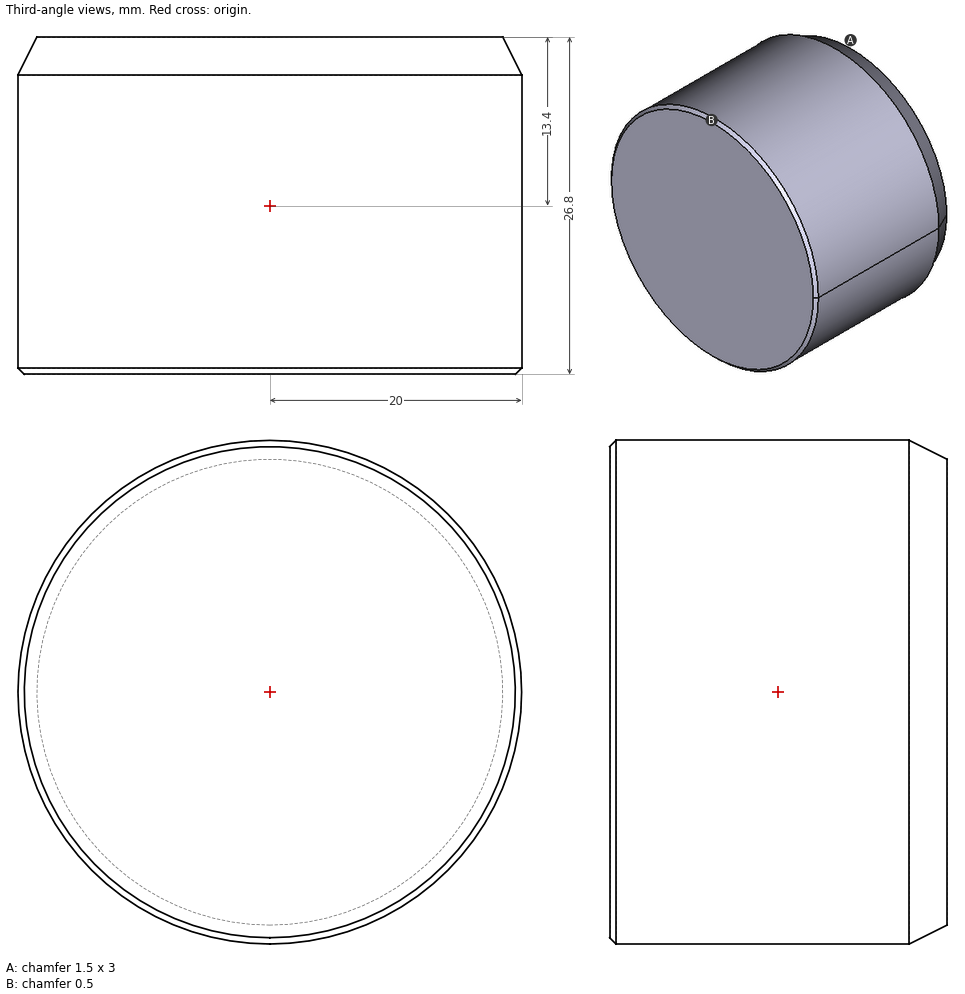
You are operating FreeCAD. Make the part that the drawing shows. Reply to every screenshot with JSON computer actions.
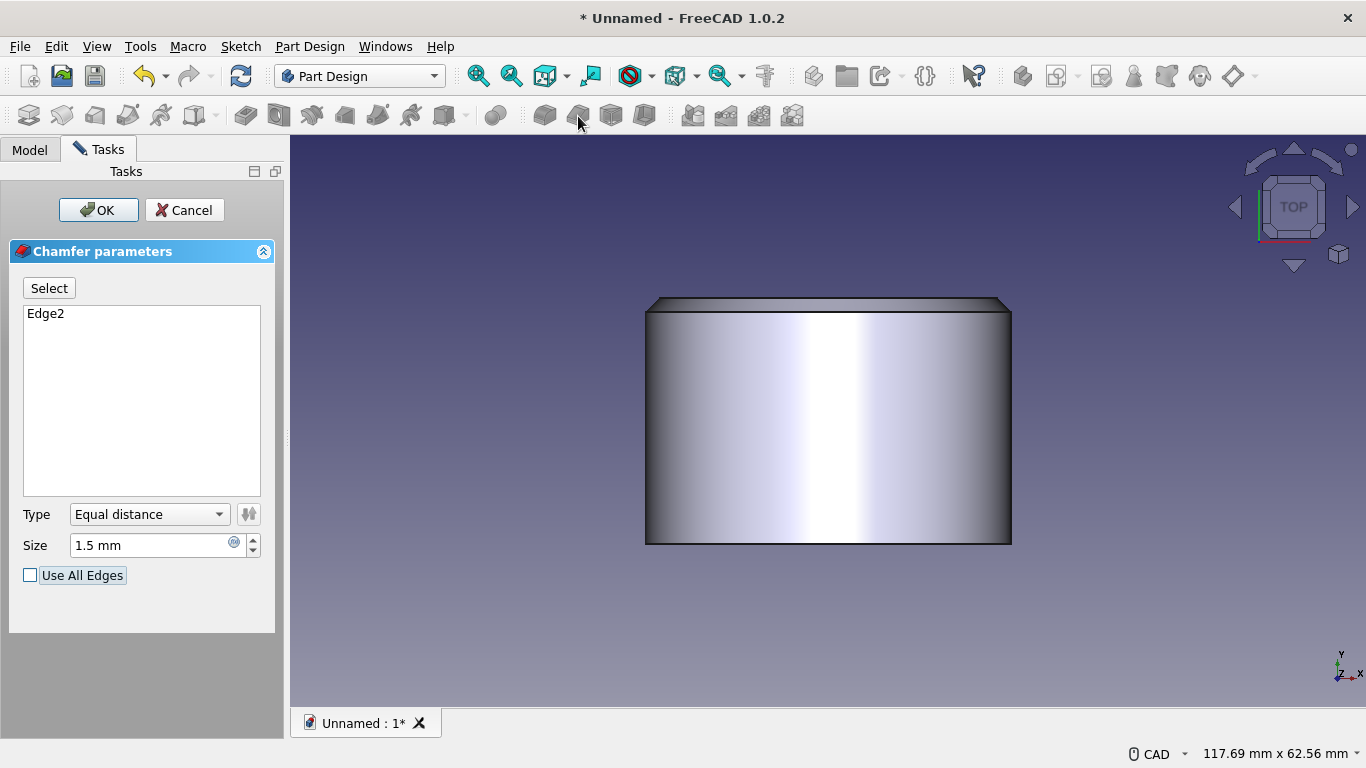
{"action": "left_click", "coordinate": [150, 514]}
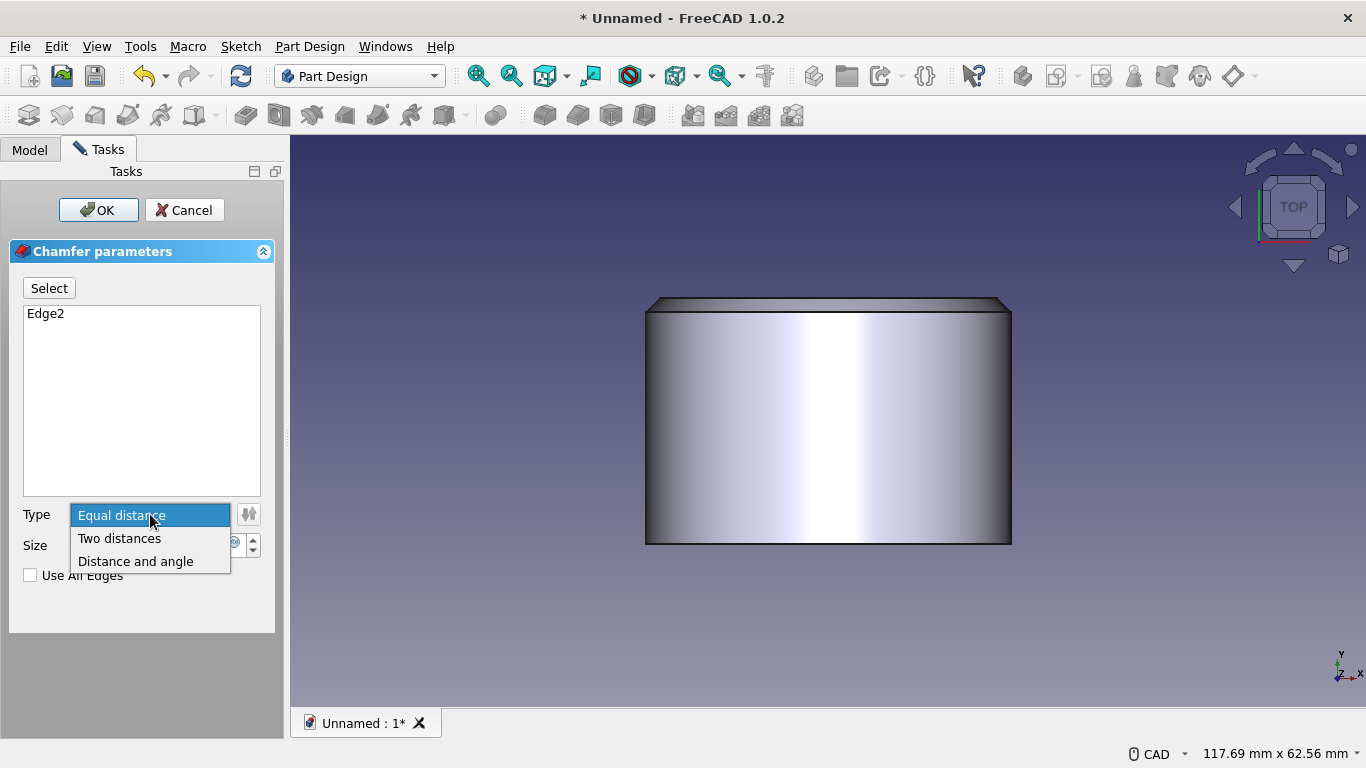
{"action": "left_click", "coordinate": [148, 538]}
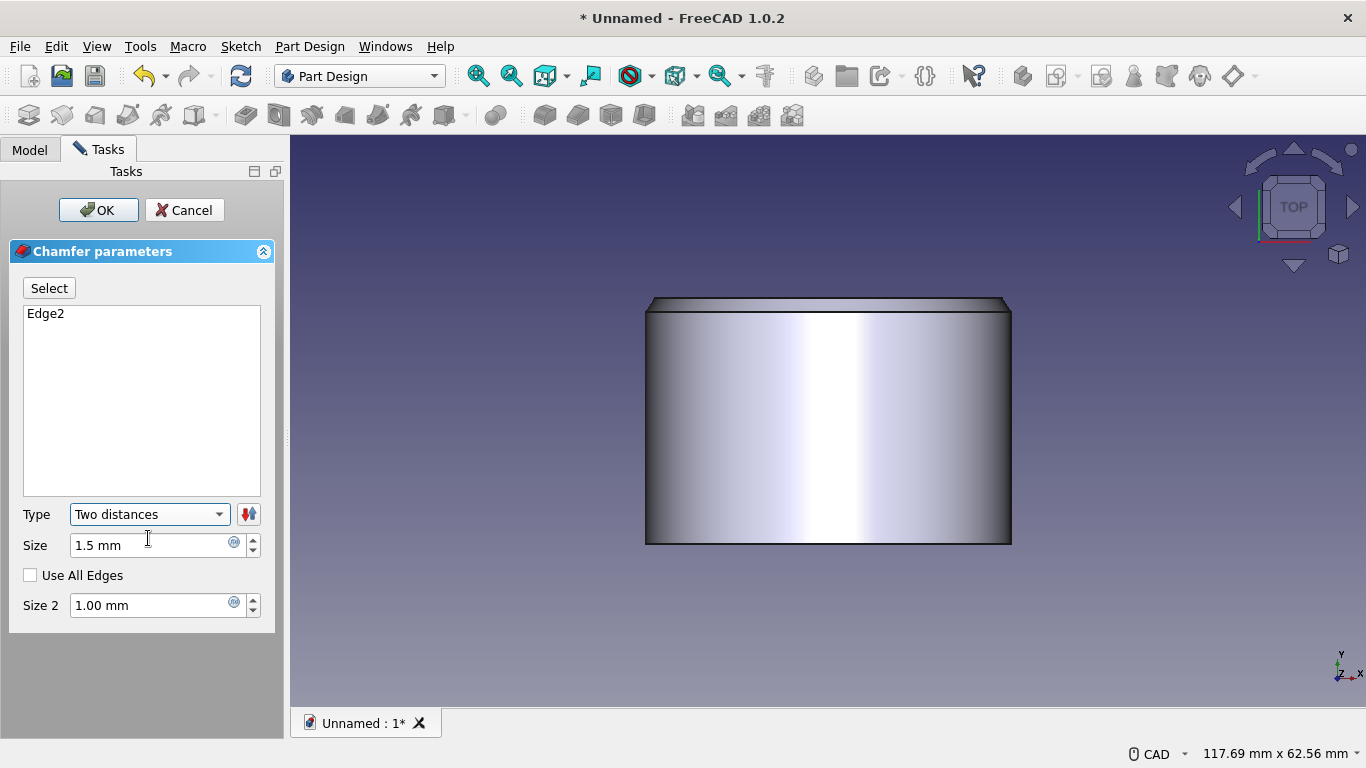
{"action": "triple_click", "coordinate": [158, 606]}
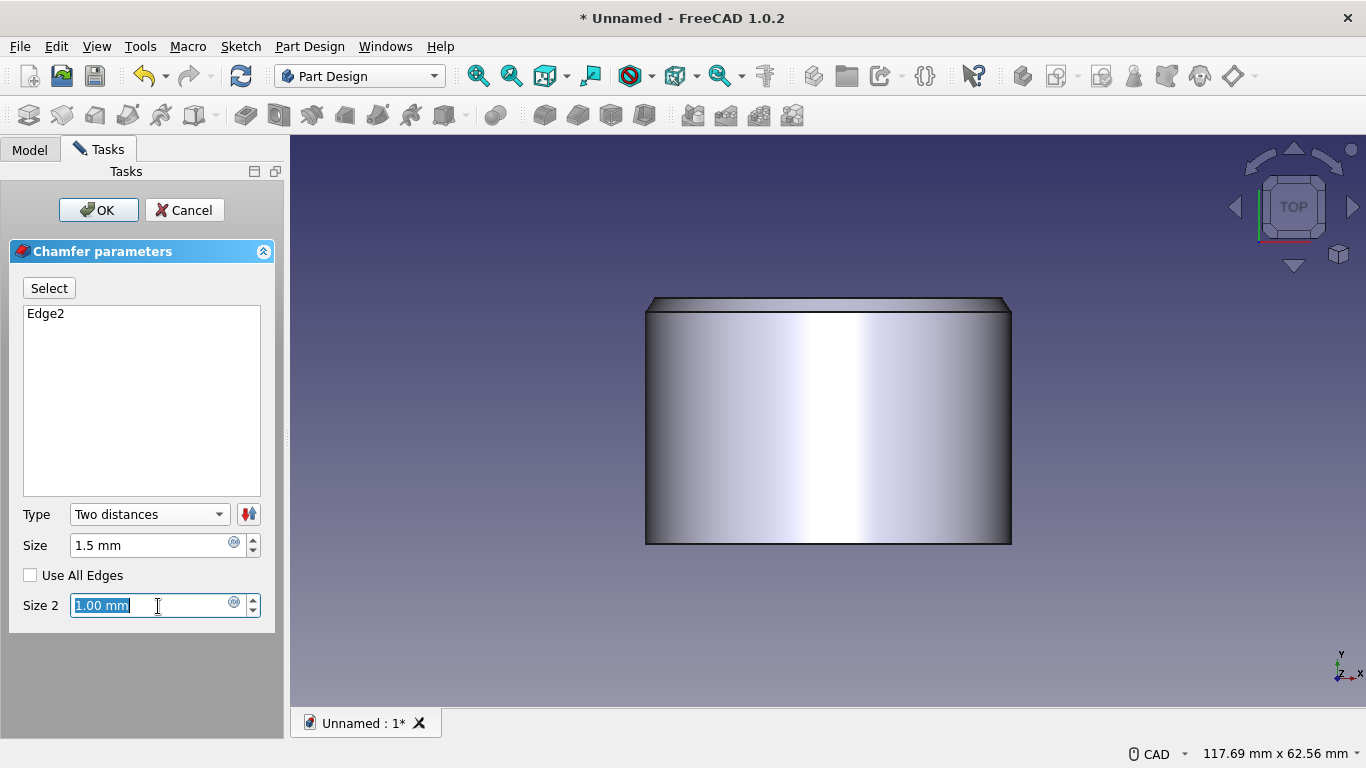
{"action": "type", "text": "3"}
{"action": "key", "text": "Tab"}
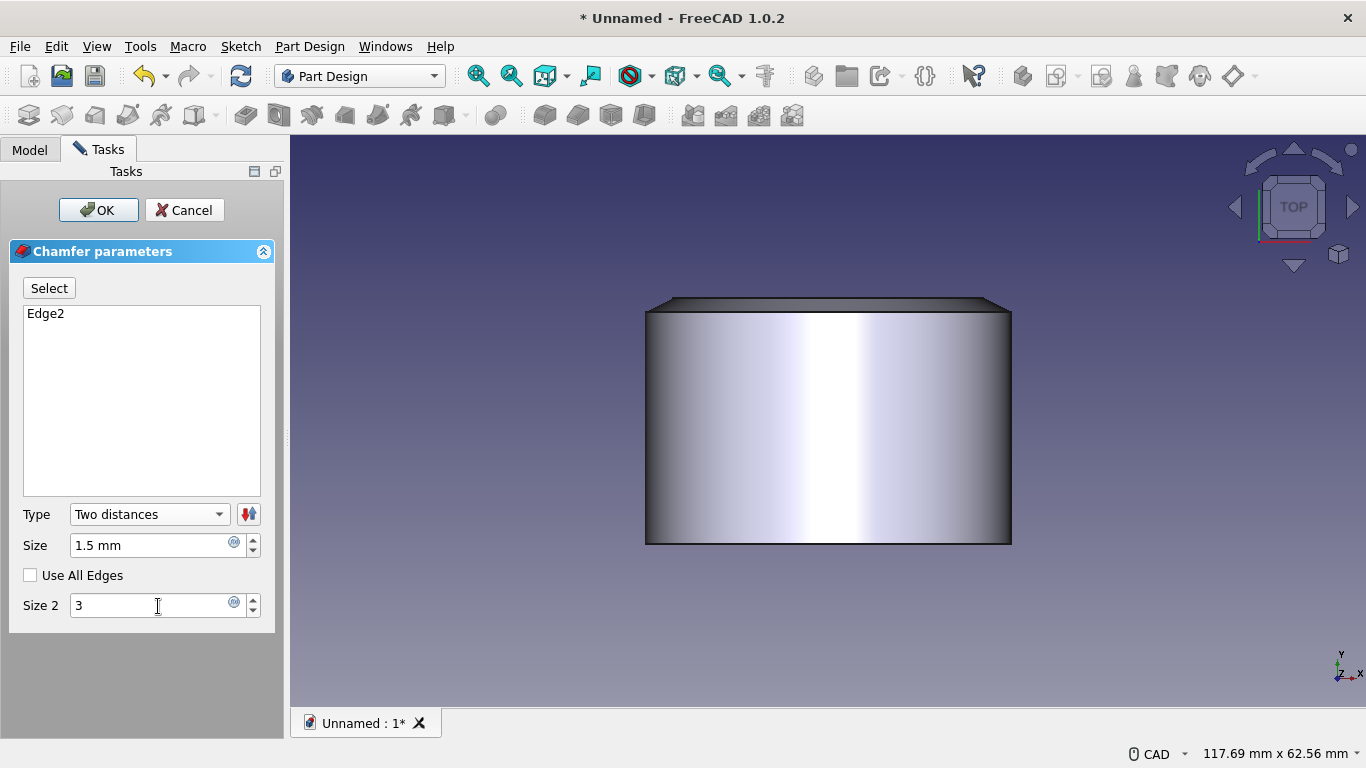
{"action": "left_click", "coordinate": [249, 514]}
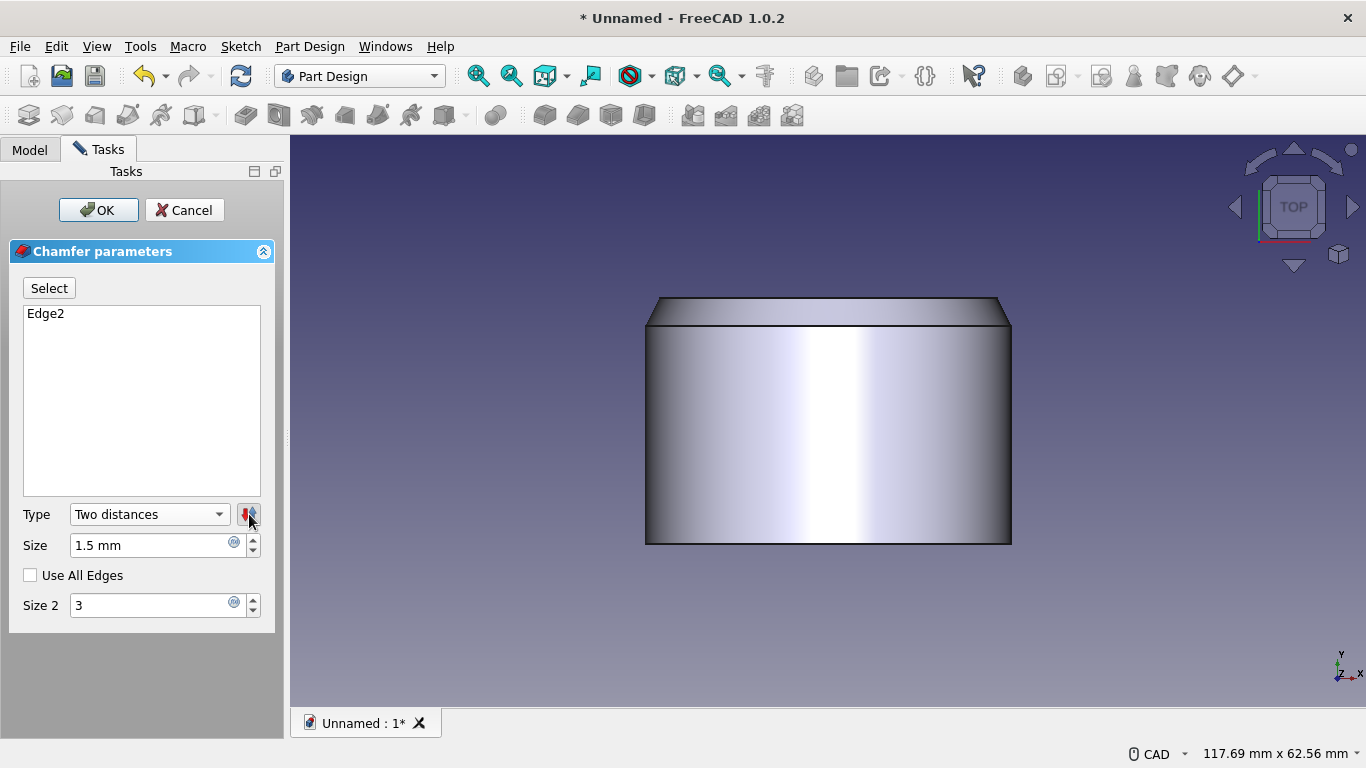
{"action": "left_click", "coordinate": [99, 210]}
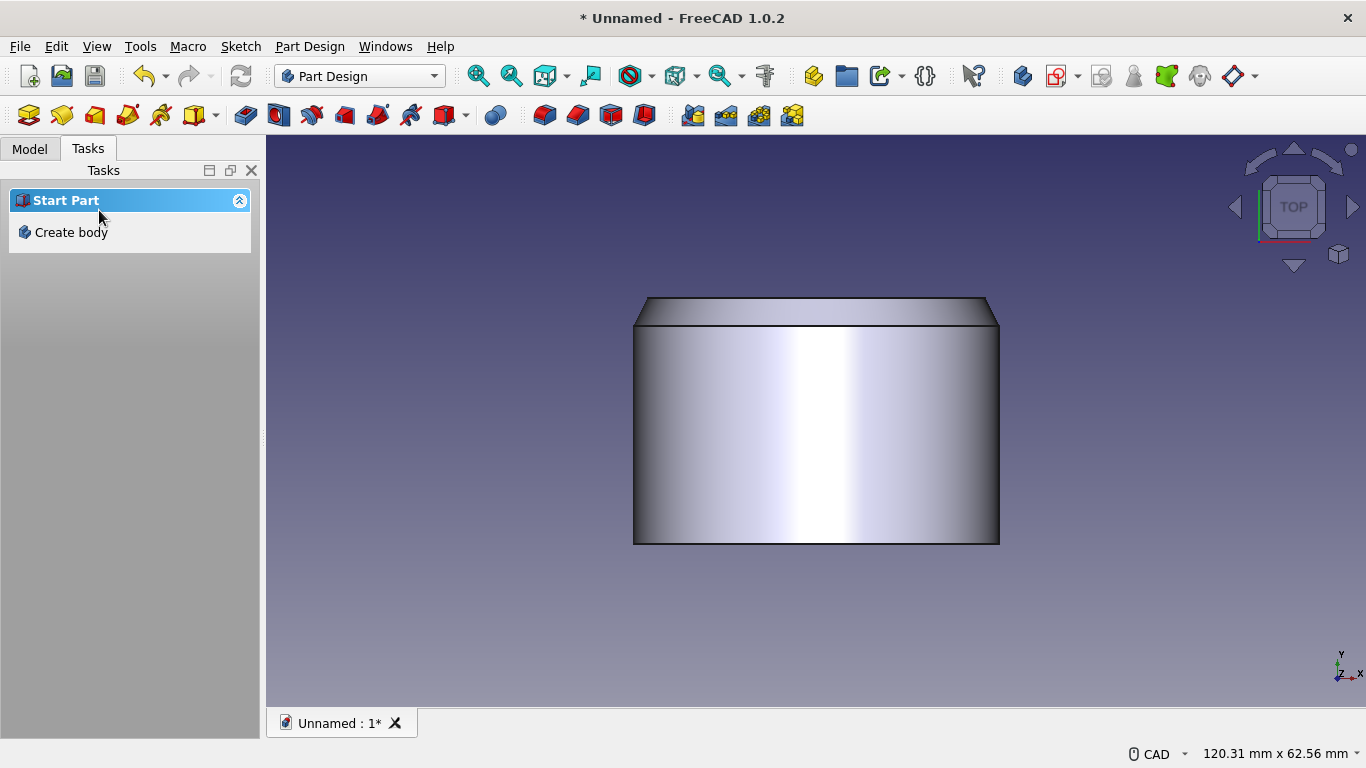
{"action": "left_click", "coordinate": [479, 76]}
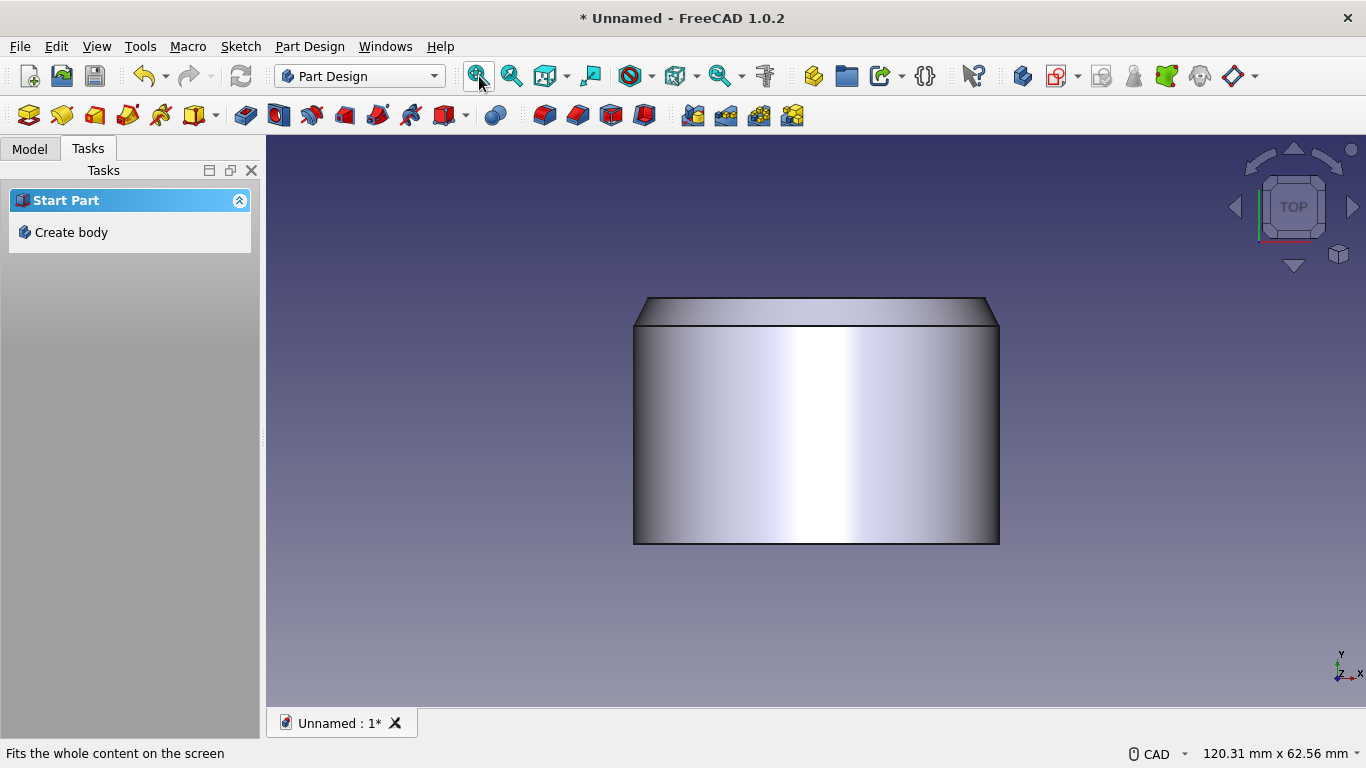
{"action": "left_click", "coordinate": [668, 543]}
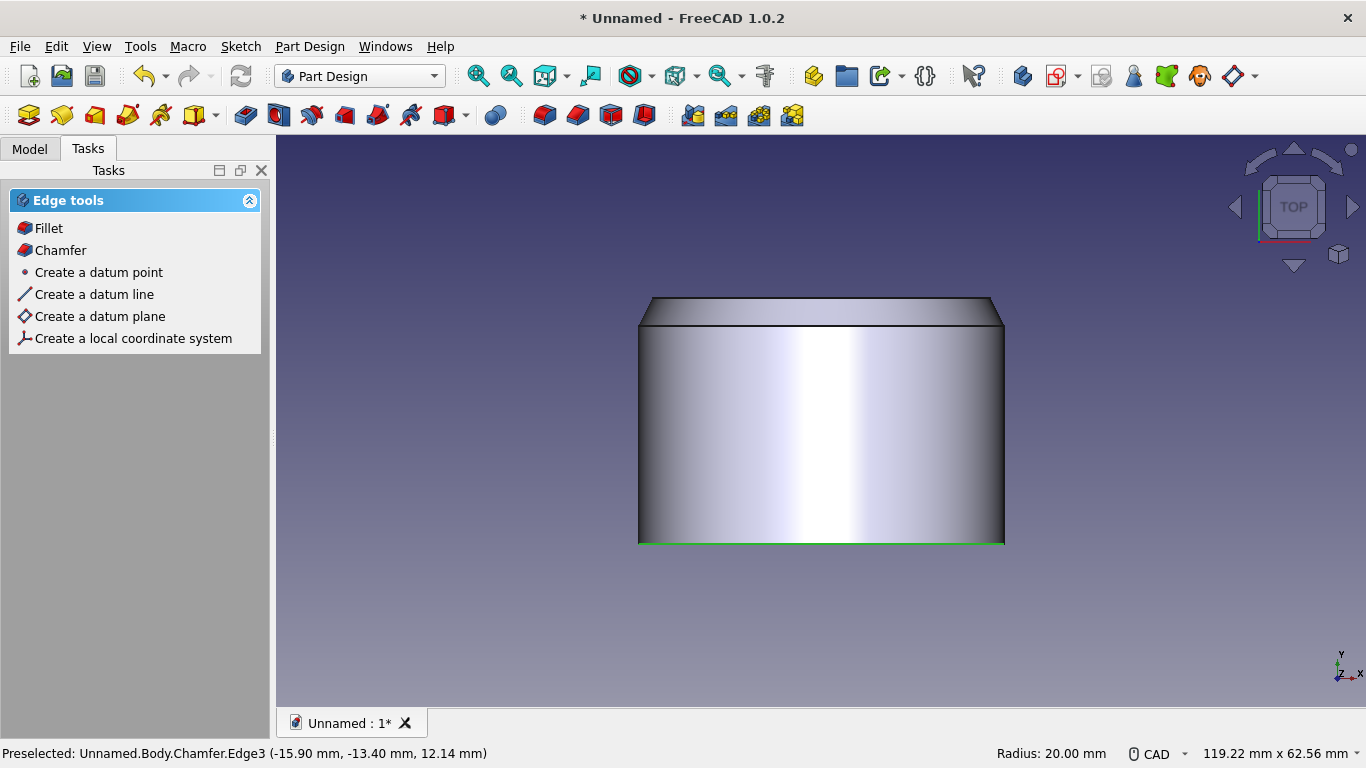
{"action": "left_click", "coordinate": [578, 116]}